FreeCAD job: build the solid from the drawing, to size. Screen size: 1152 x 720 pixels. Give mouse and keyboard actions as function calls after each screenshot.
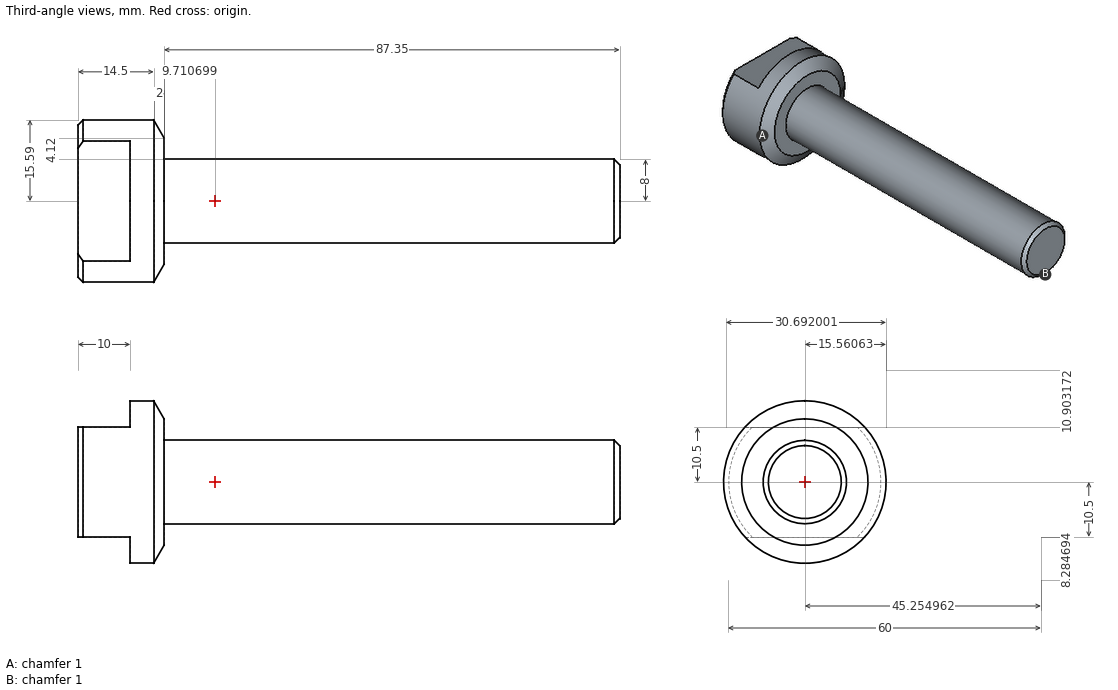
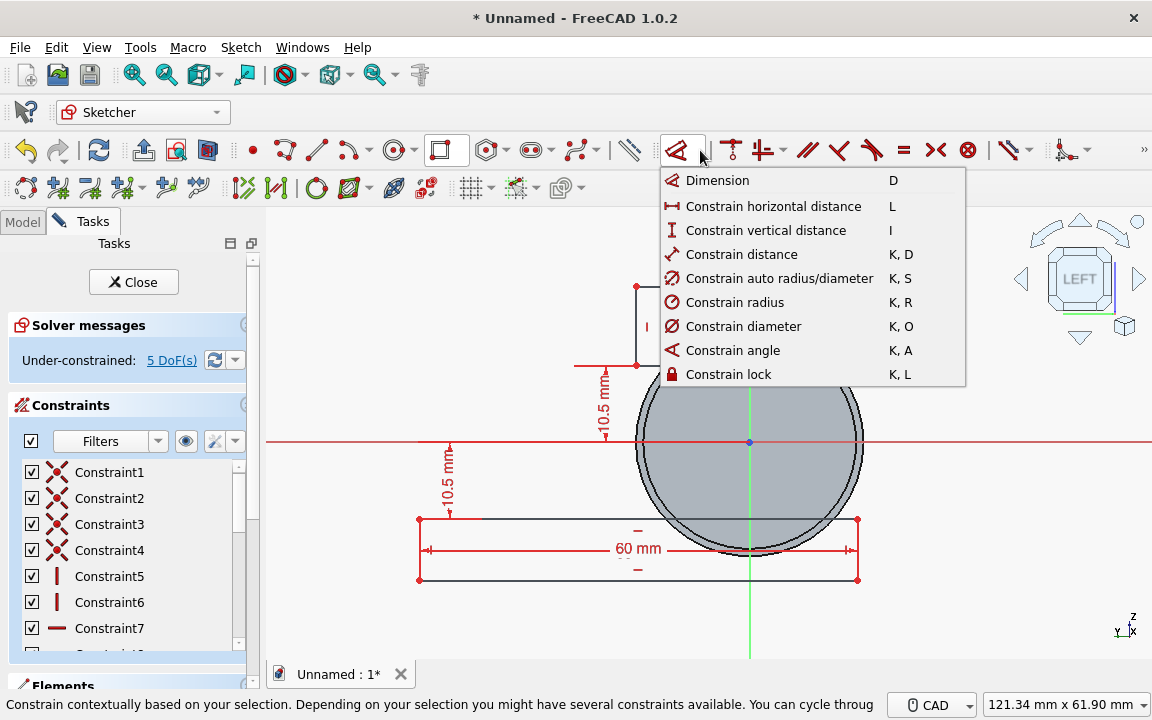
click(813, 230)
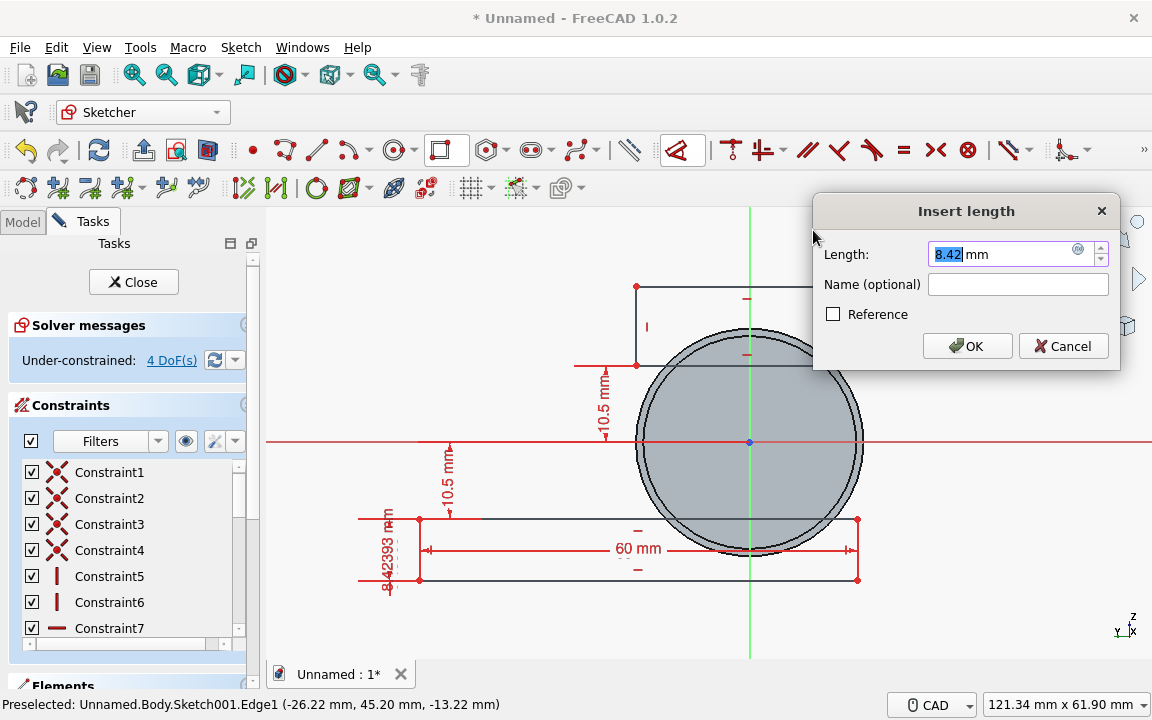
text(8.284694)
key(Return)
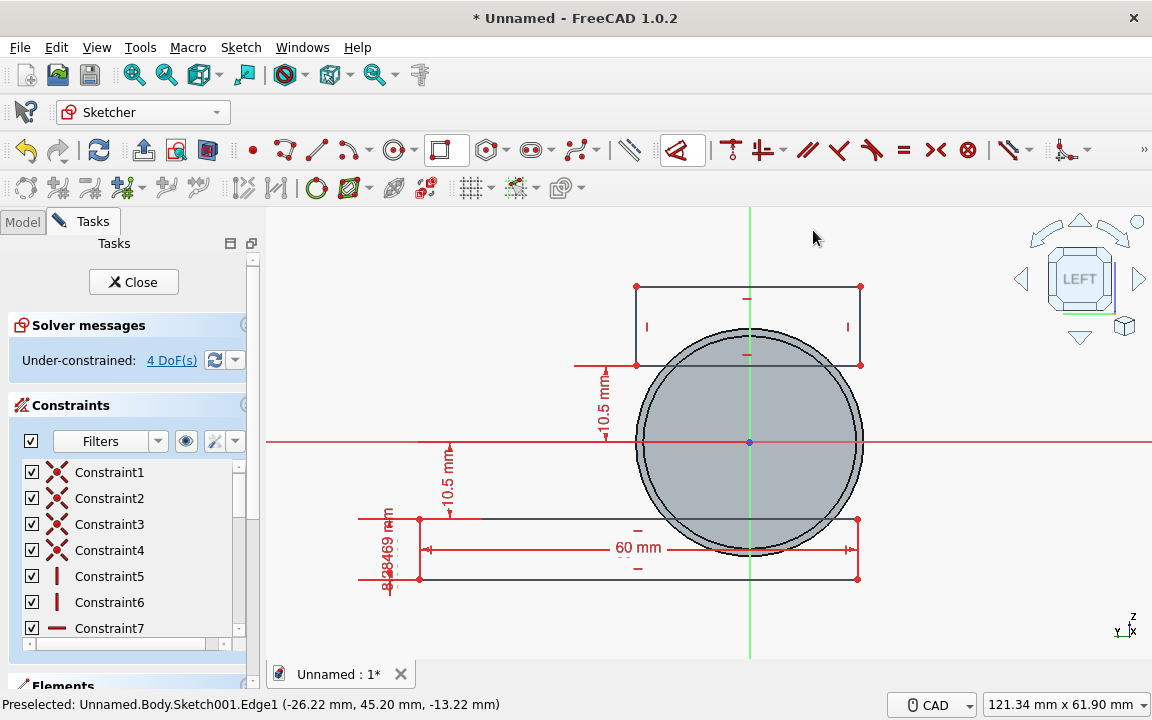
click(636, 311)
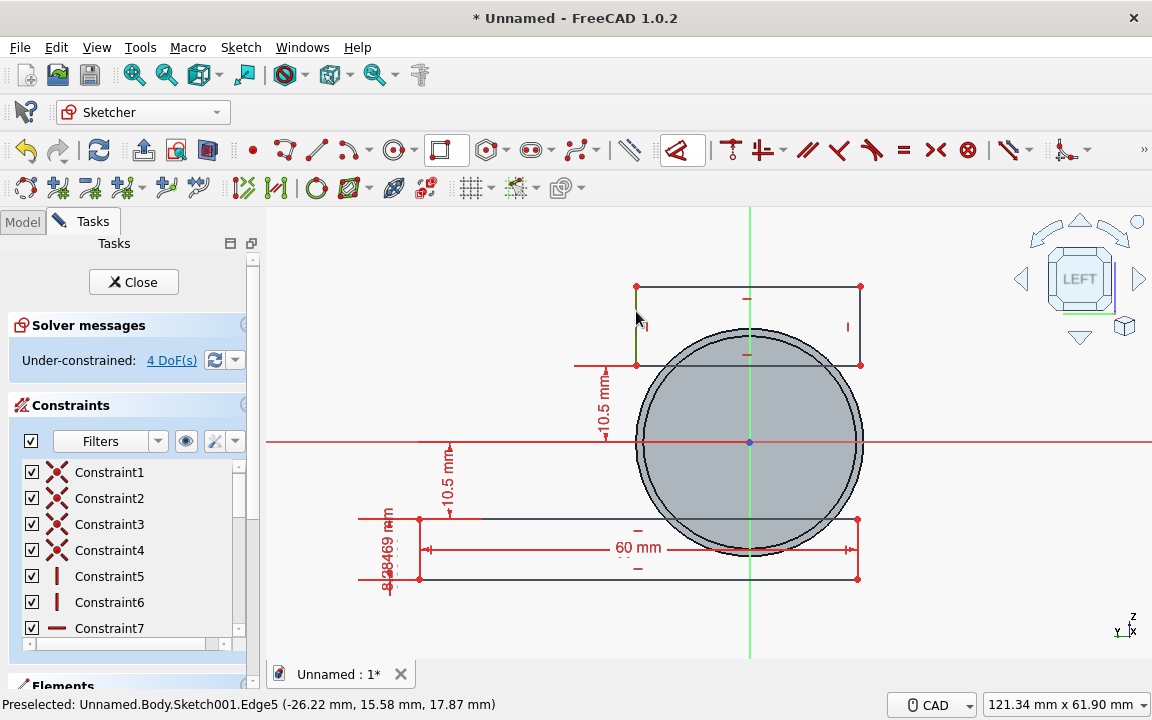
click(700, 150)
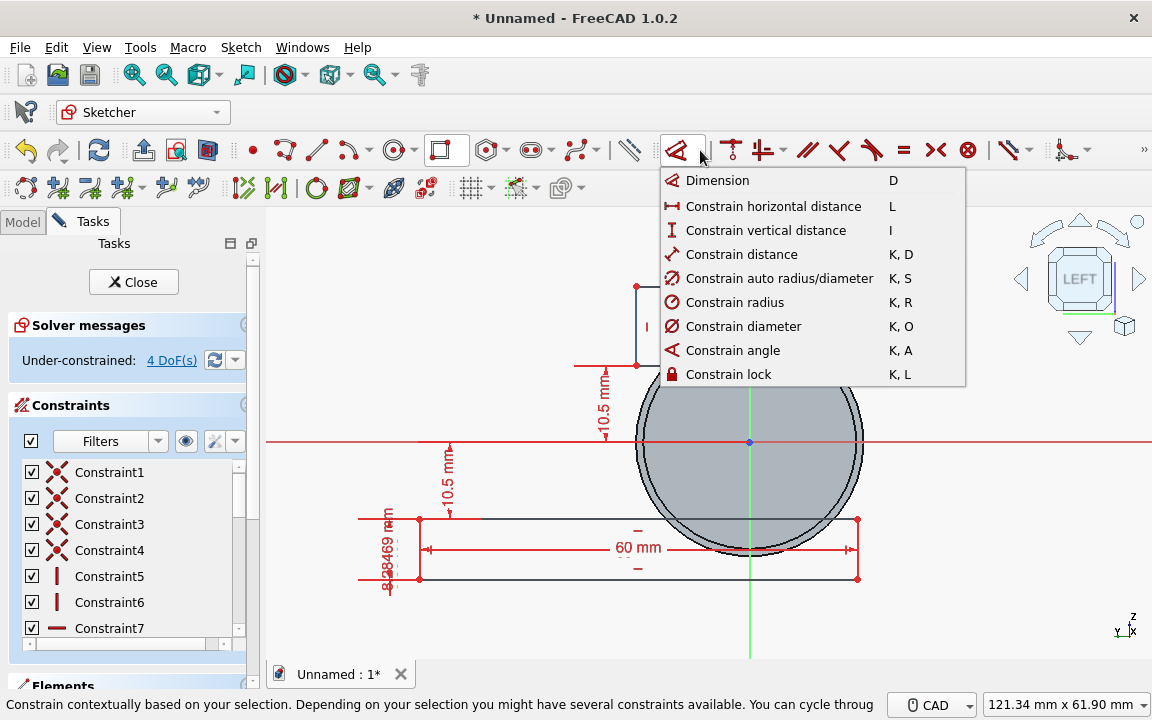
click(813, 230)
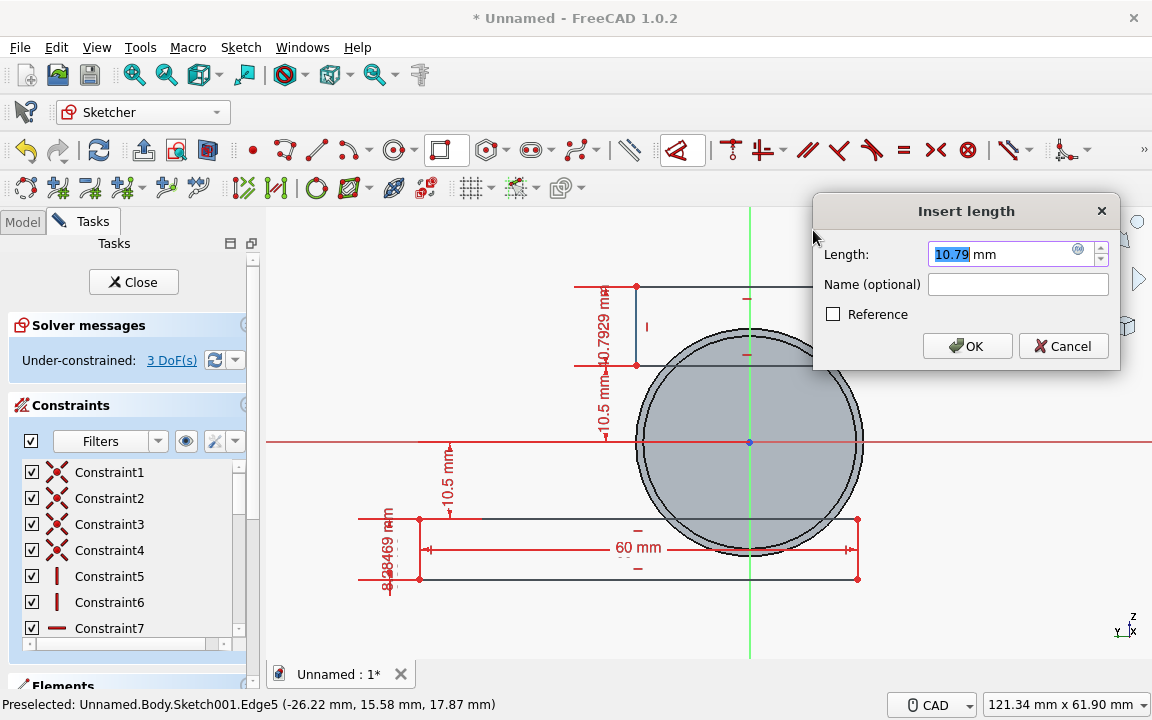
text(10.903172)
key(Return)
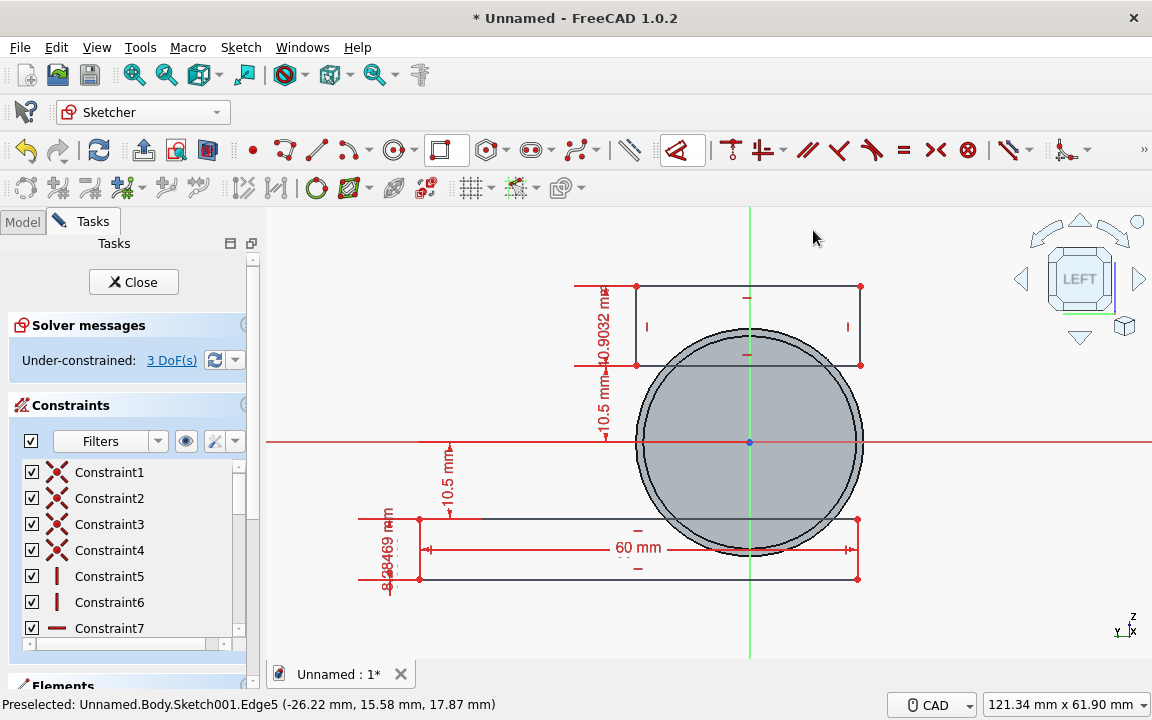
click(703, 366)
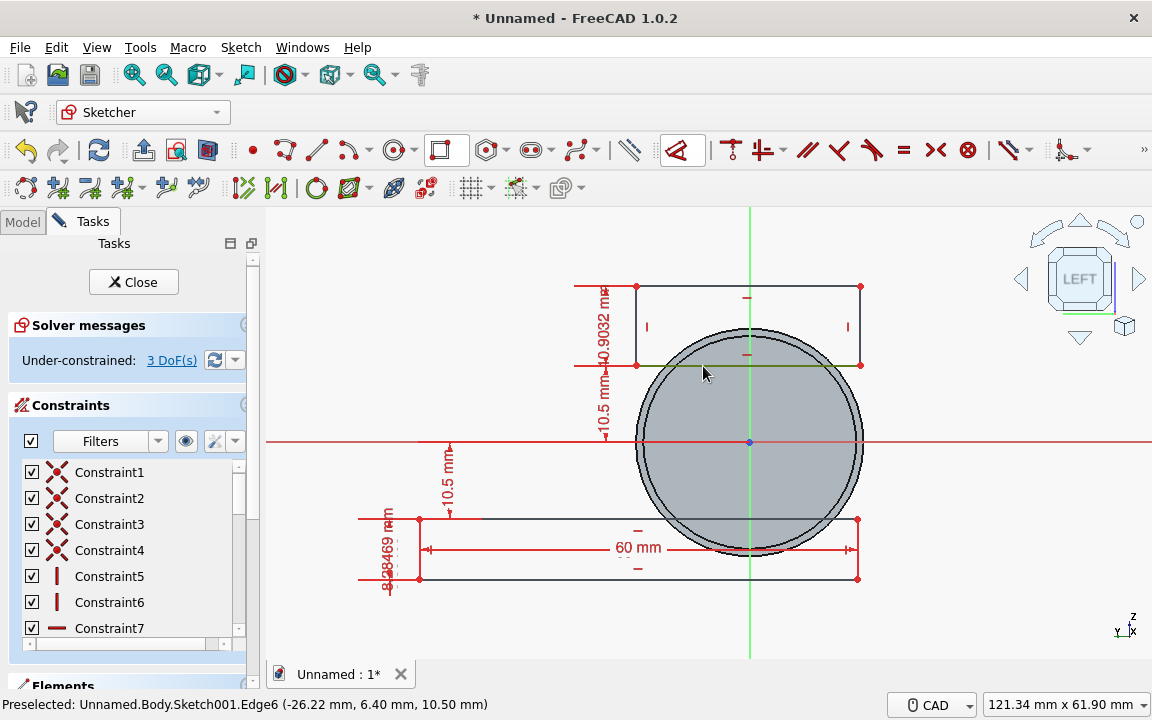
click(700, 150)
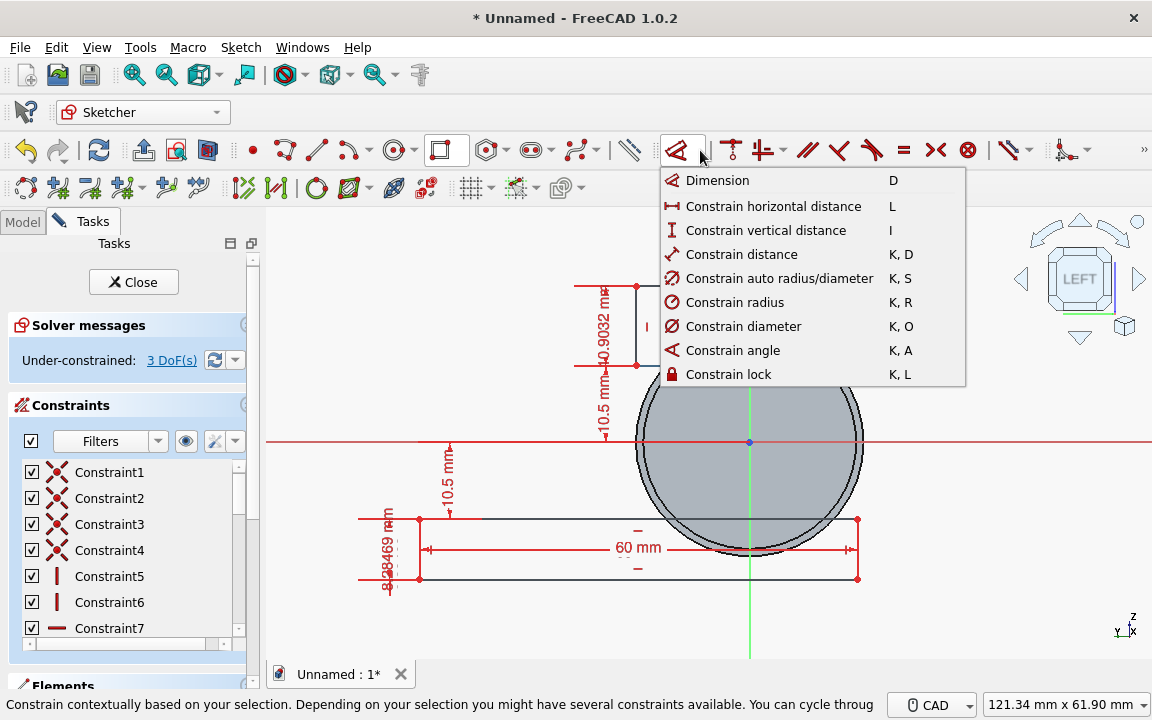
click(813, 206)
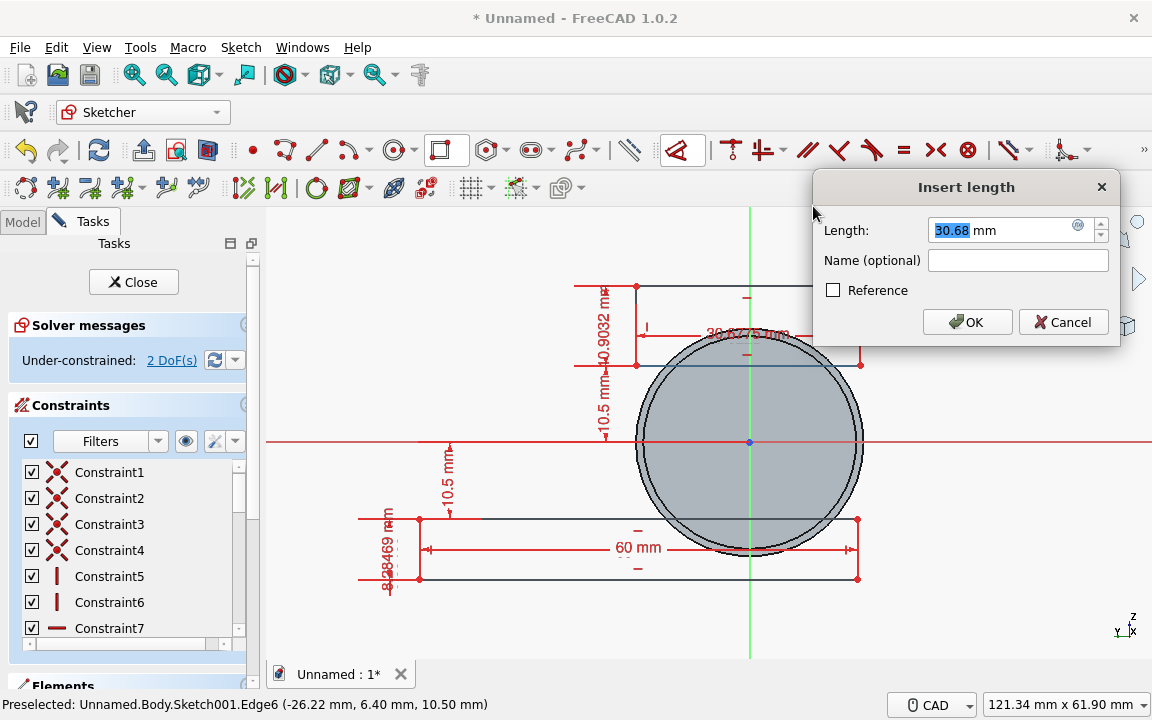
text(30.692001)
key(Return)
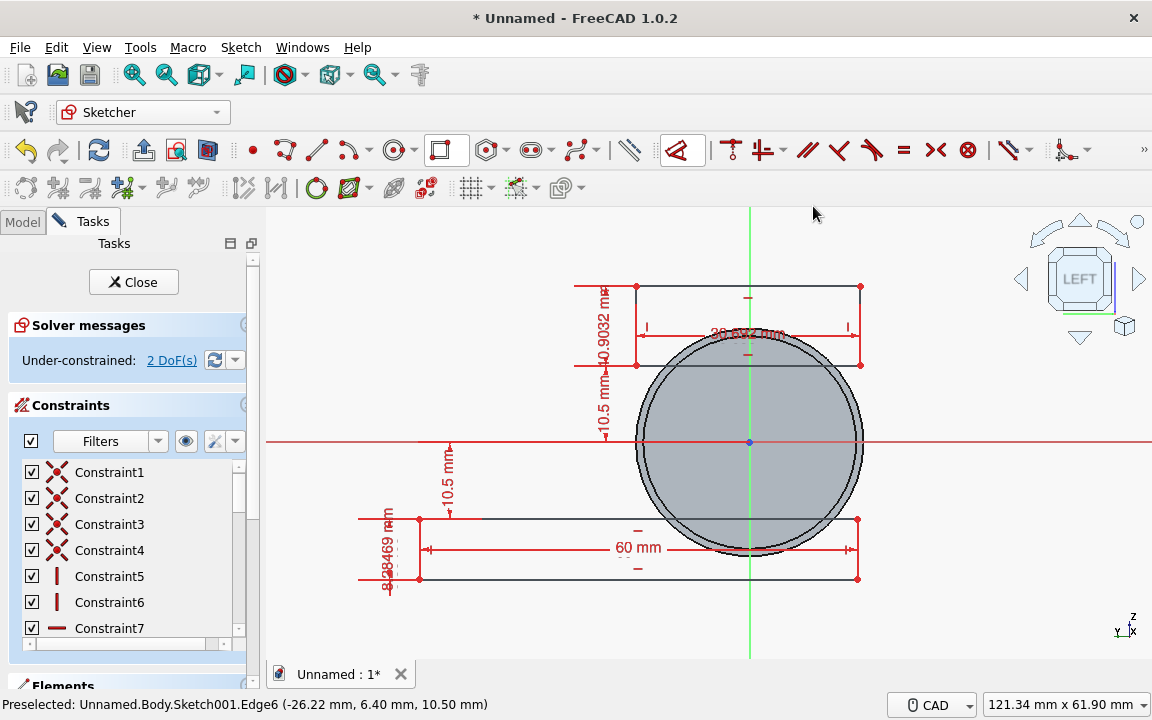
click(636, 286)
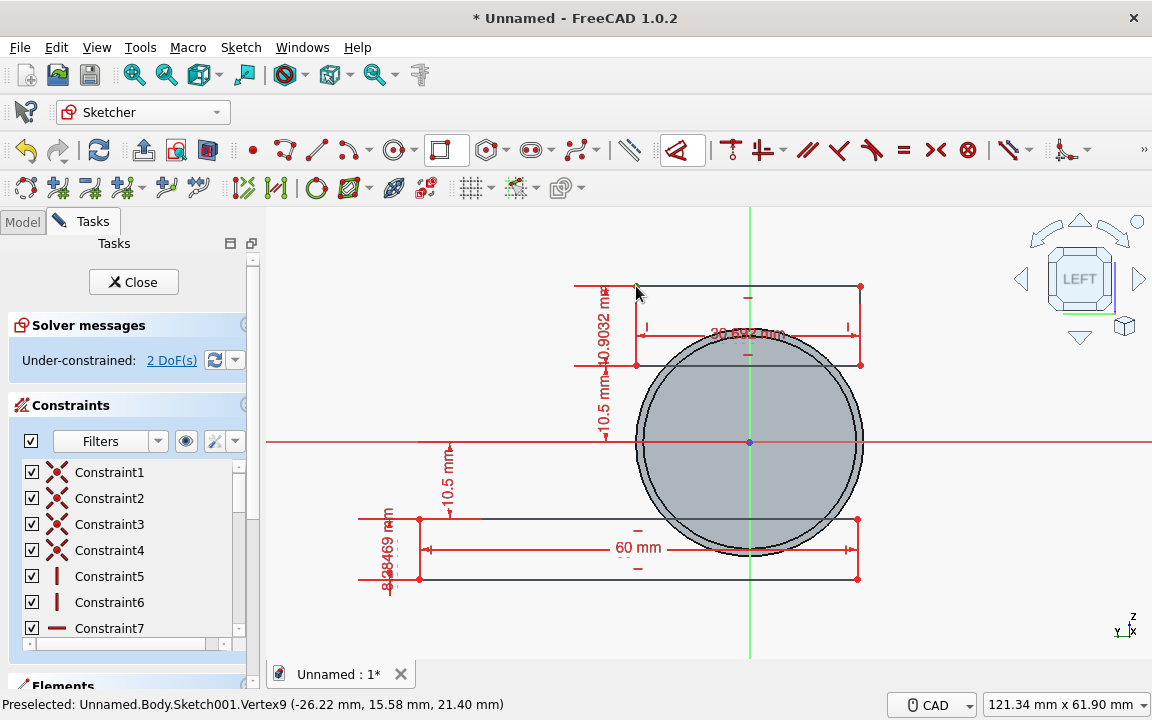
click(700, 150)